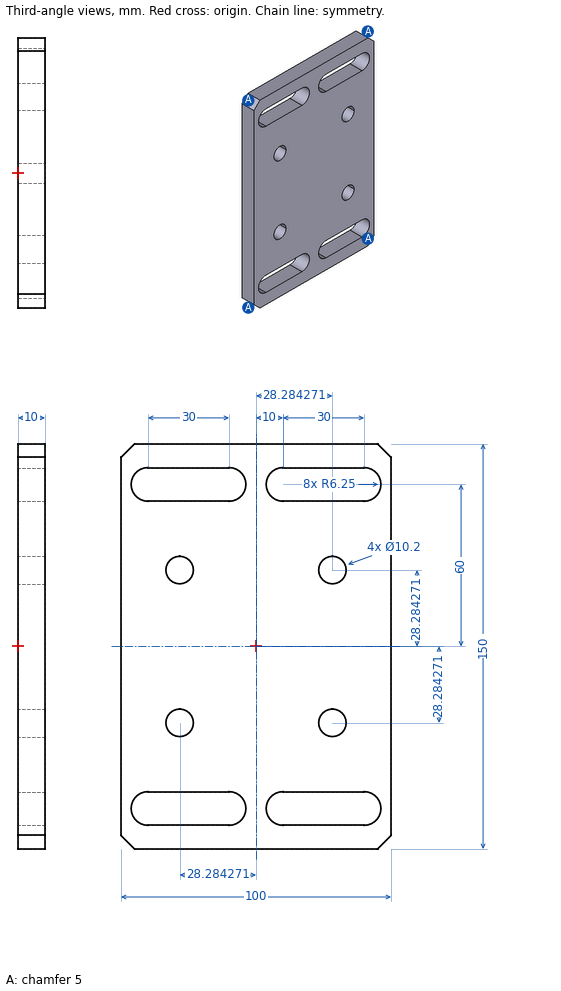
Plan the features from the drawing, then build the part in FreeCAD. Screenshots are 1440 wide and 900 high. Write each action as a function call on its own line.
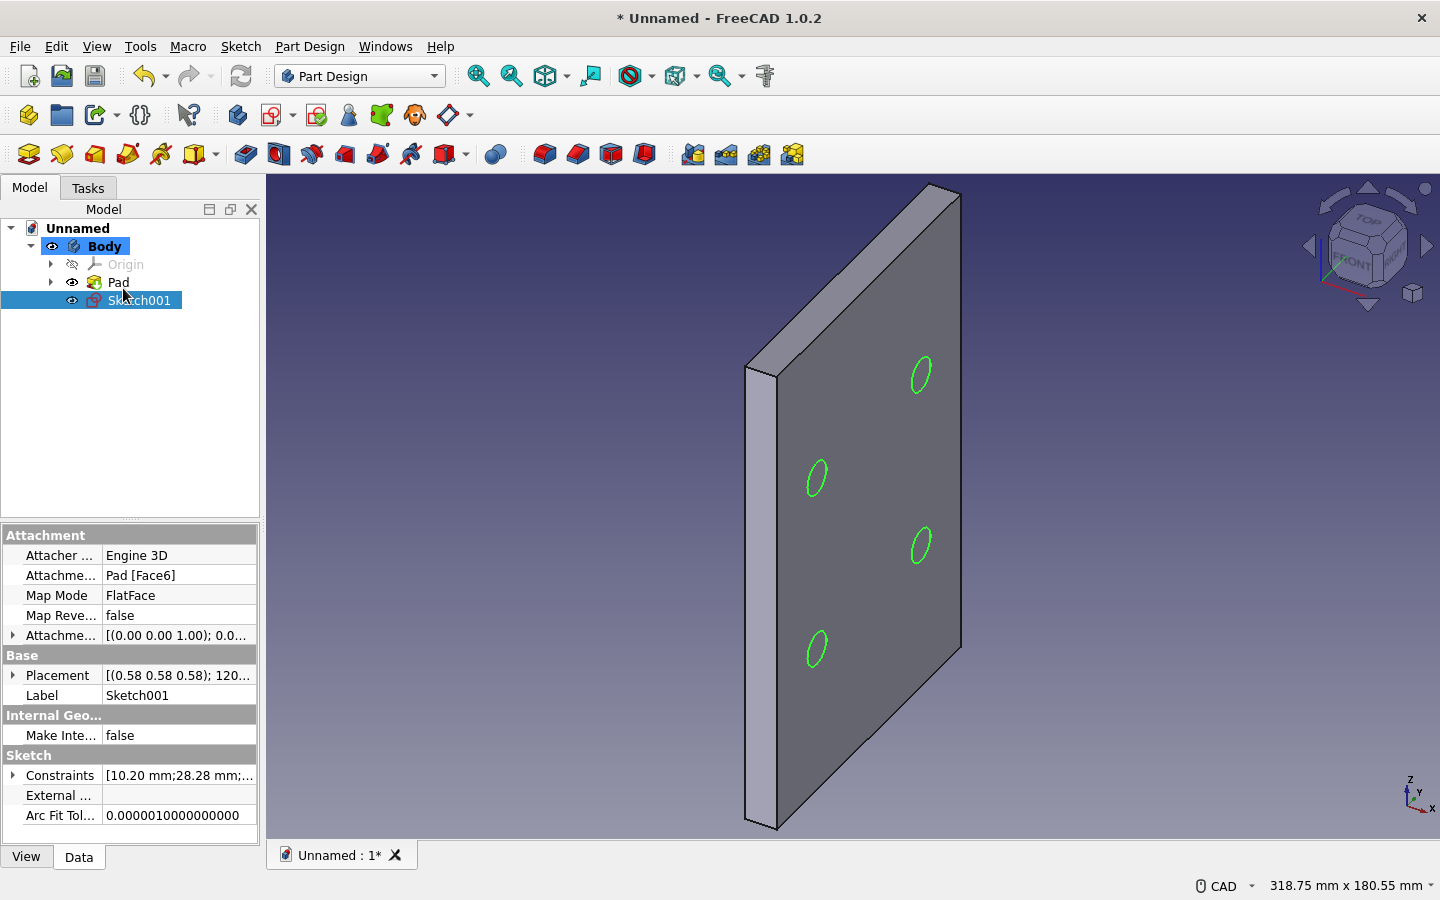
click(246, 154)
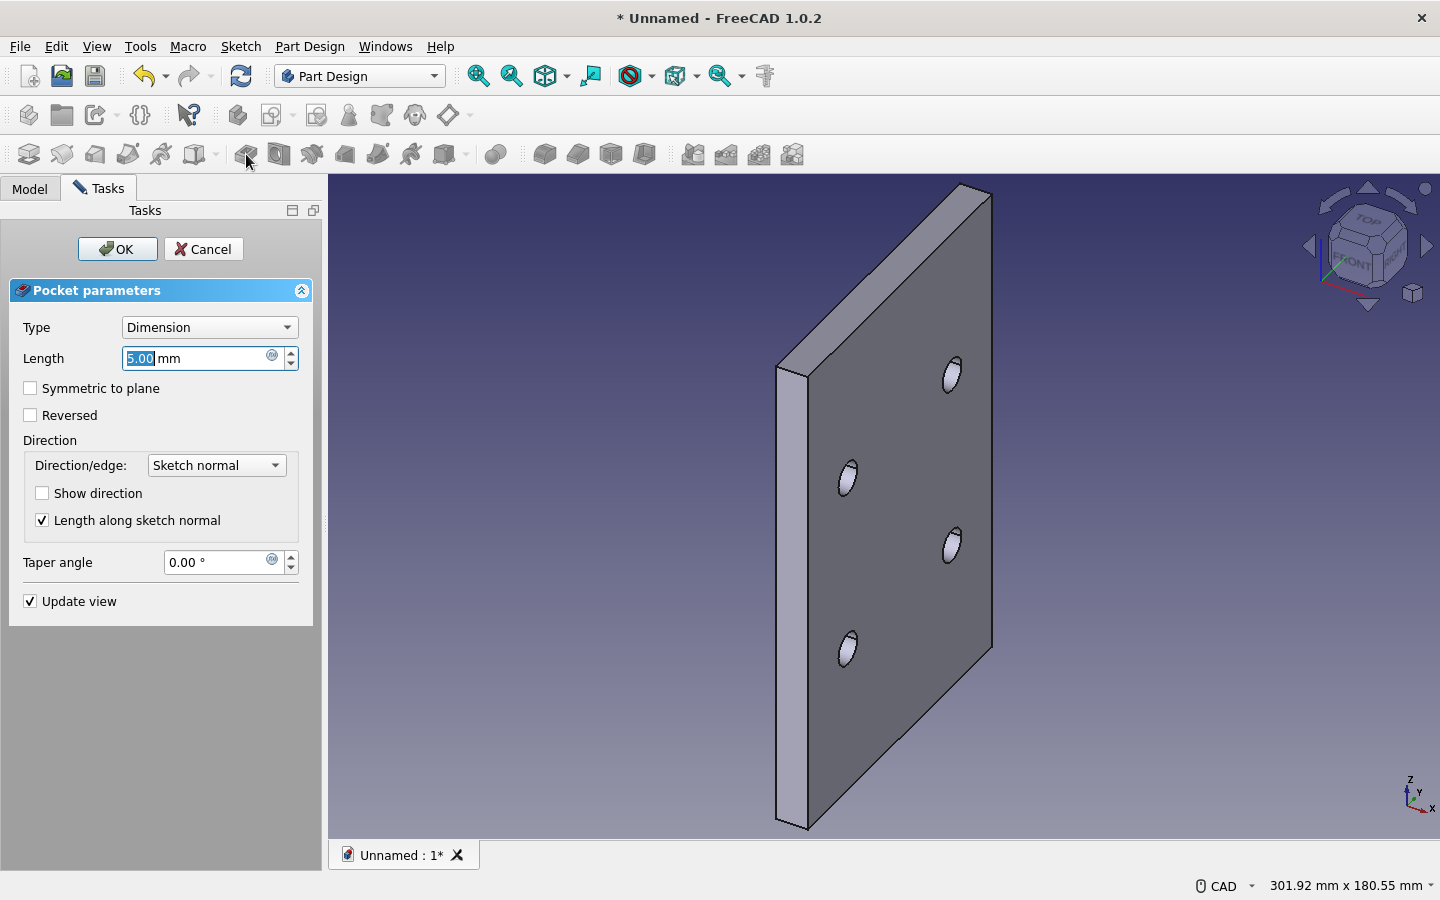
click(210, 328)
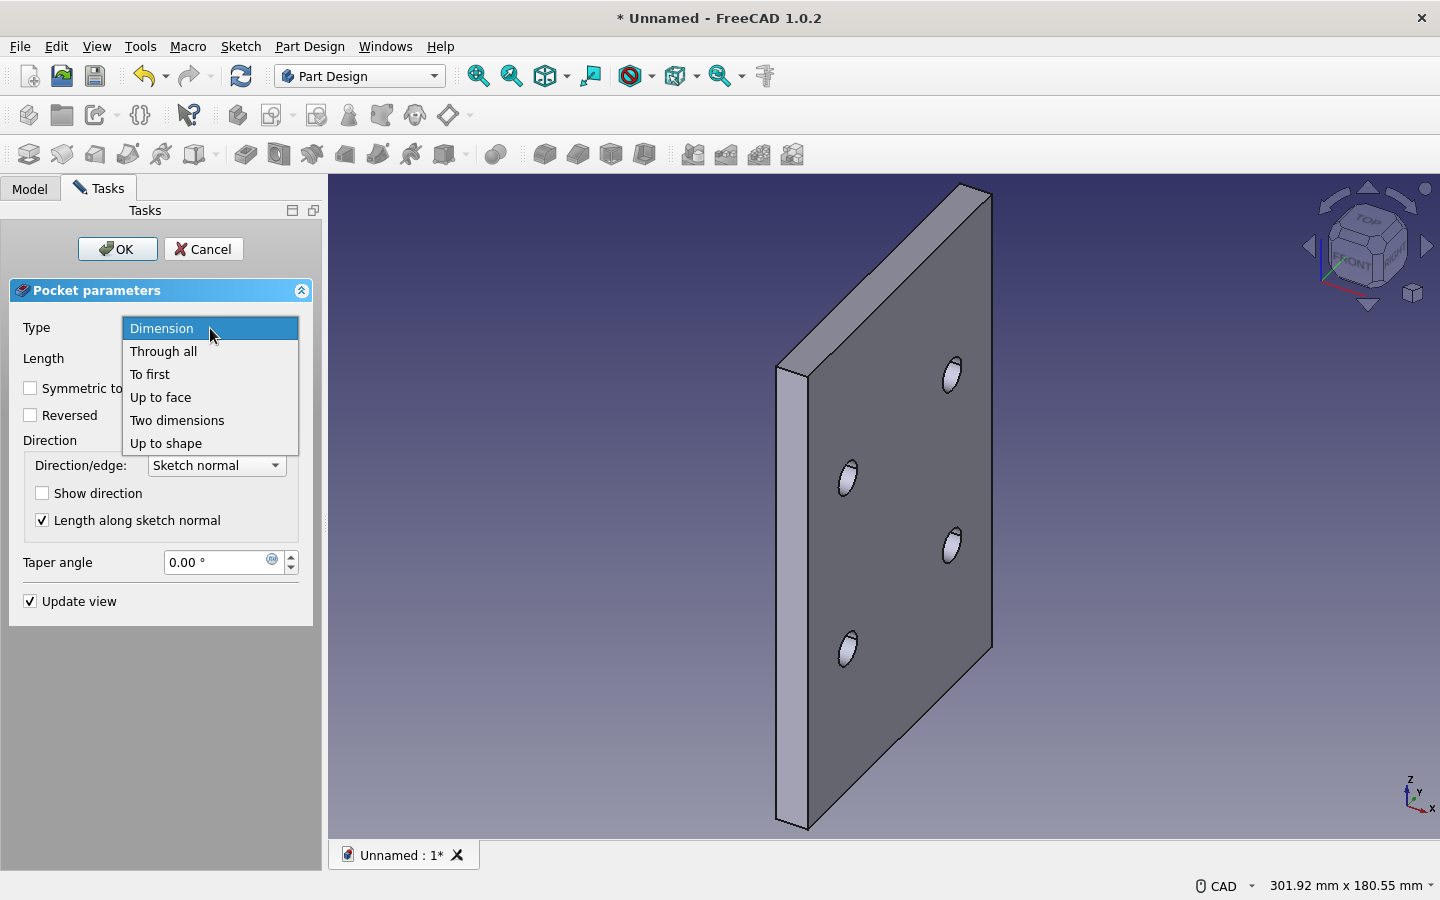
click(208, 352)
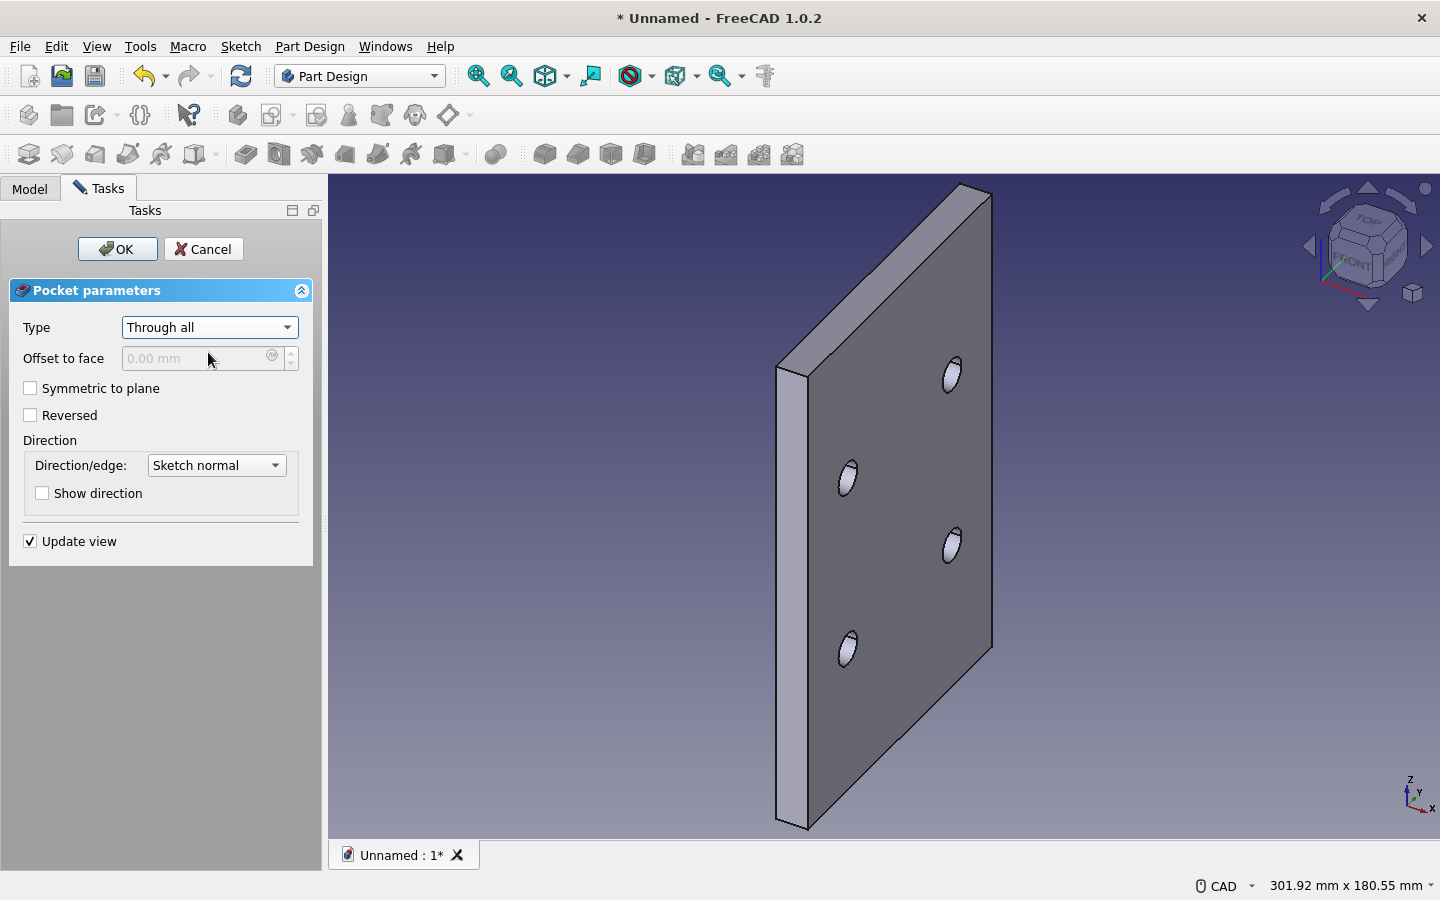
click(118, 249)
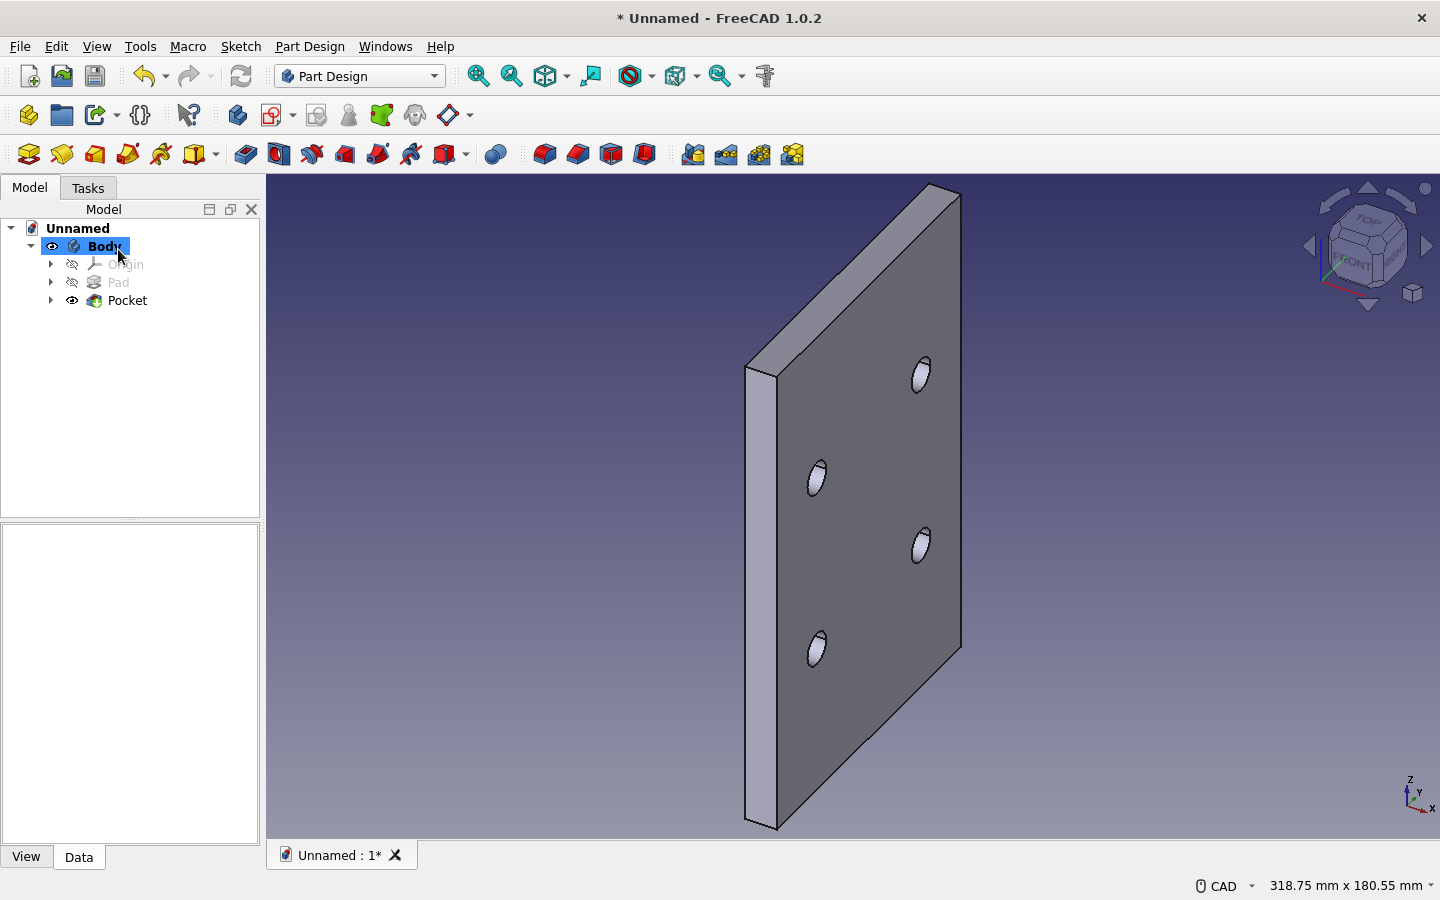
click(869, 511)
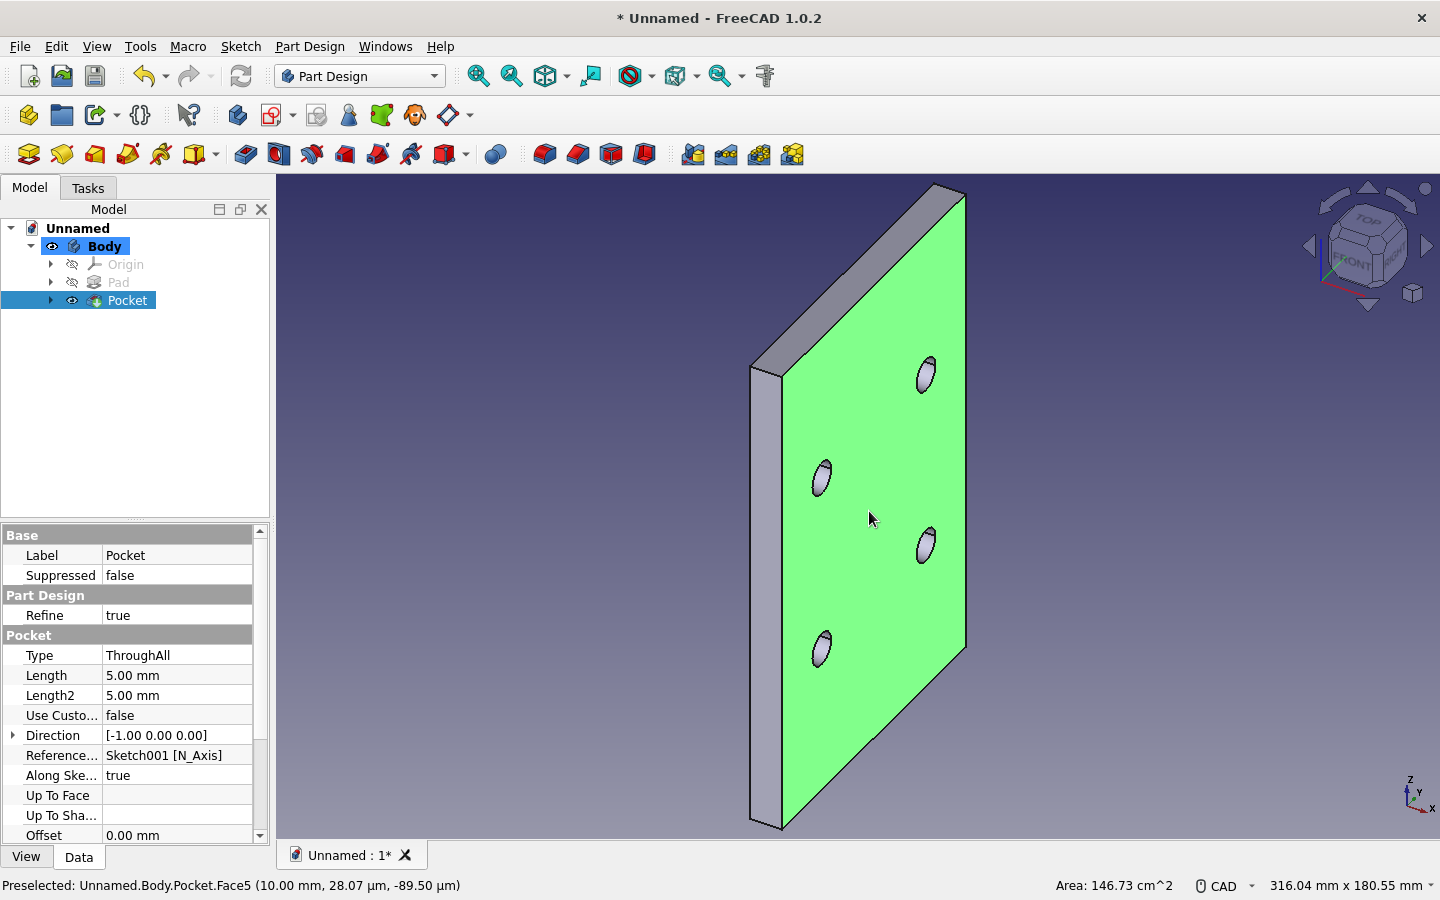
click(270, 116)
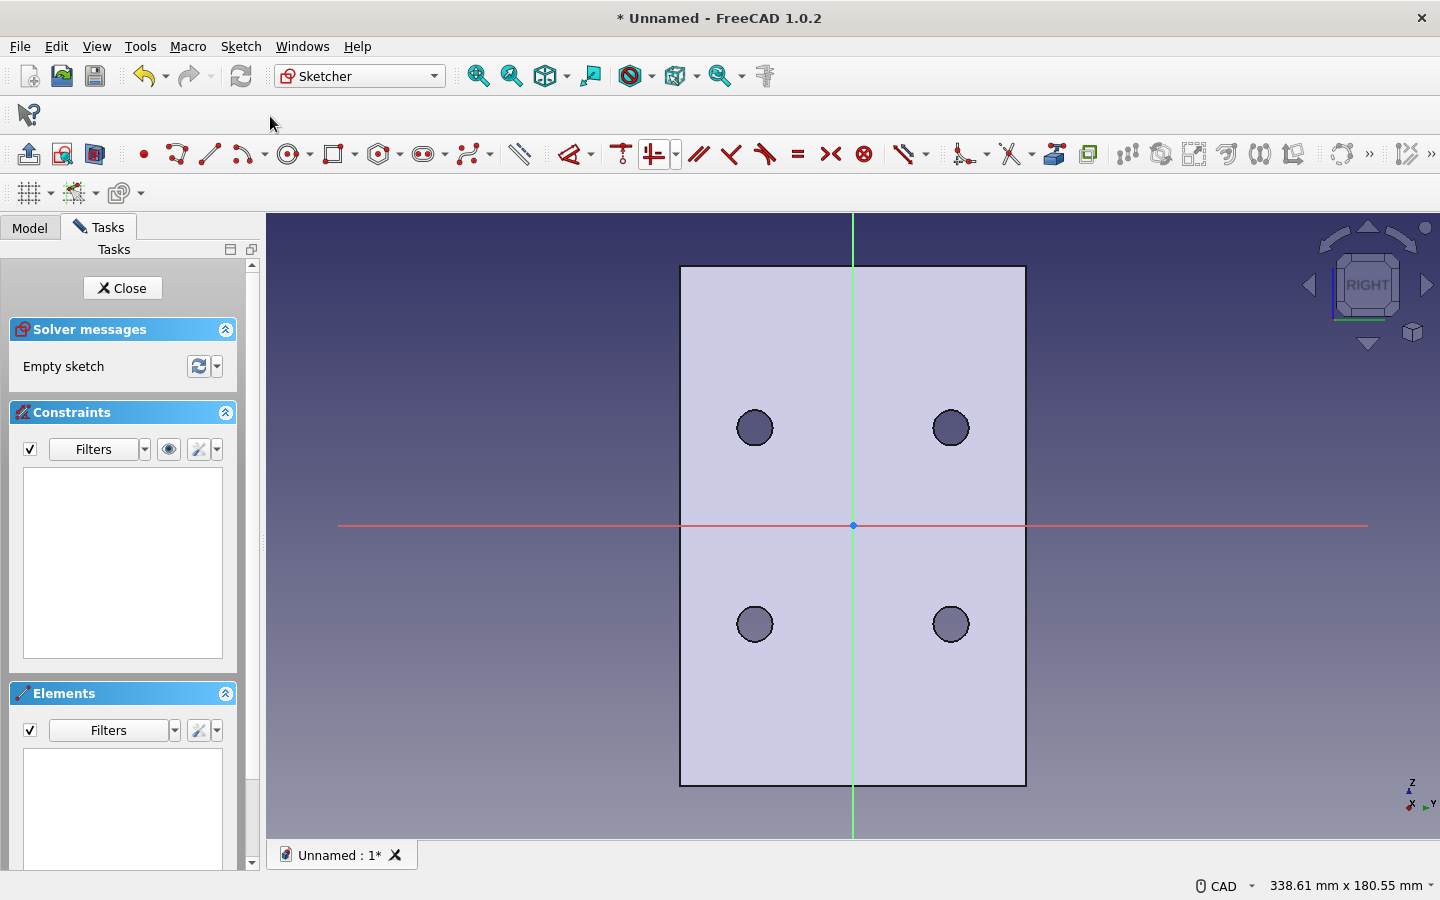
click(422, 154)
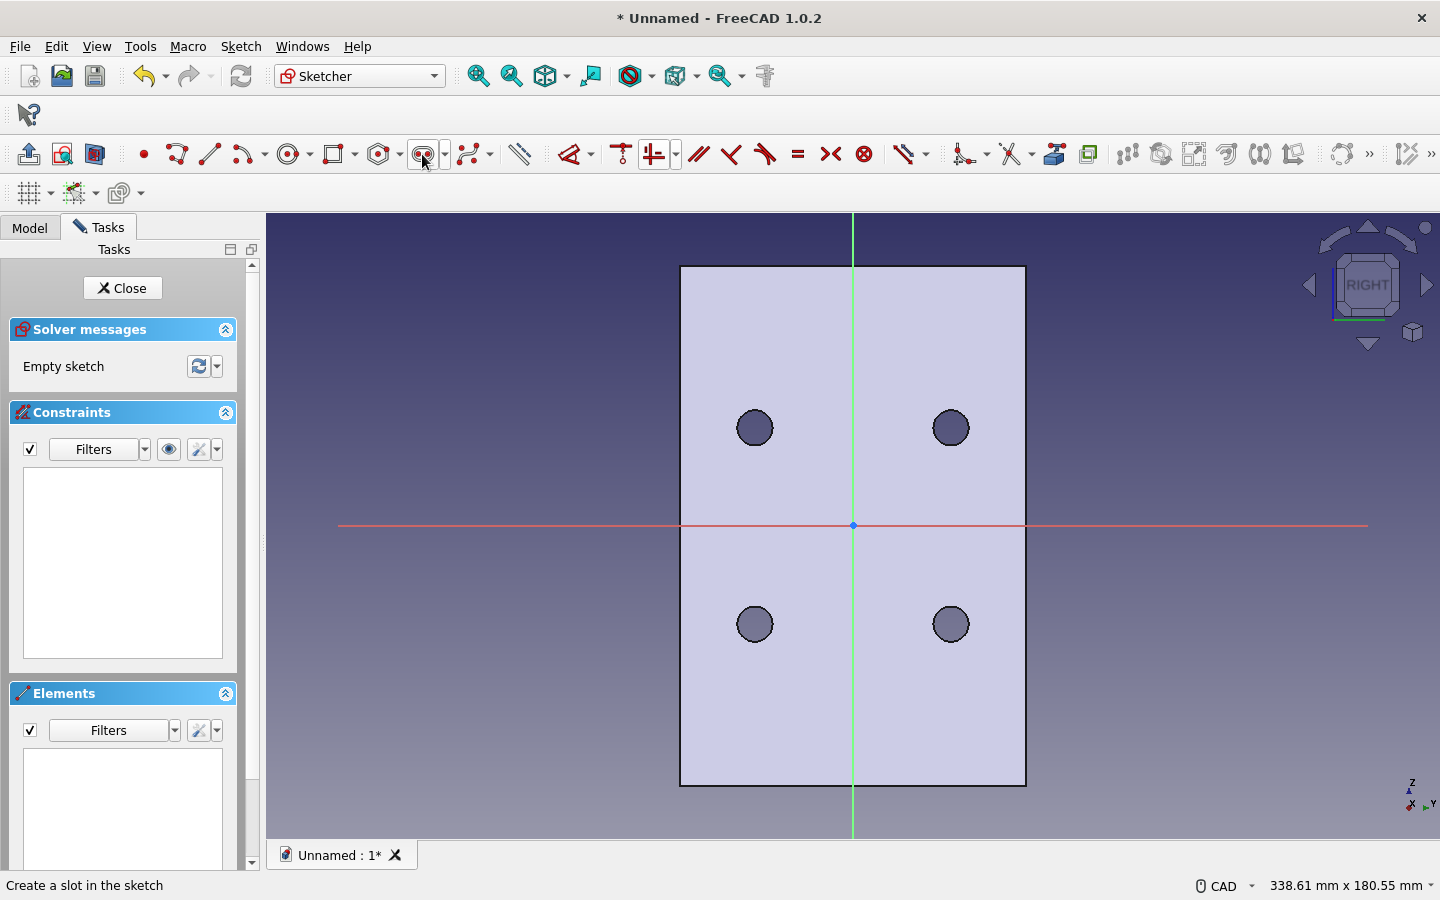
click(888, 318)